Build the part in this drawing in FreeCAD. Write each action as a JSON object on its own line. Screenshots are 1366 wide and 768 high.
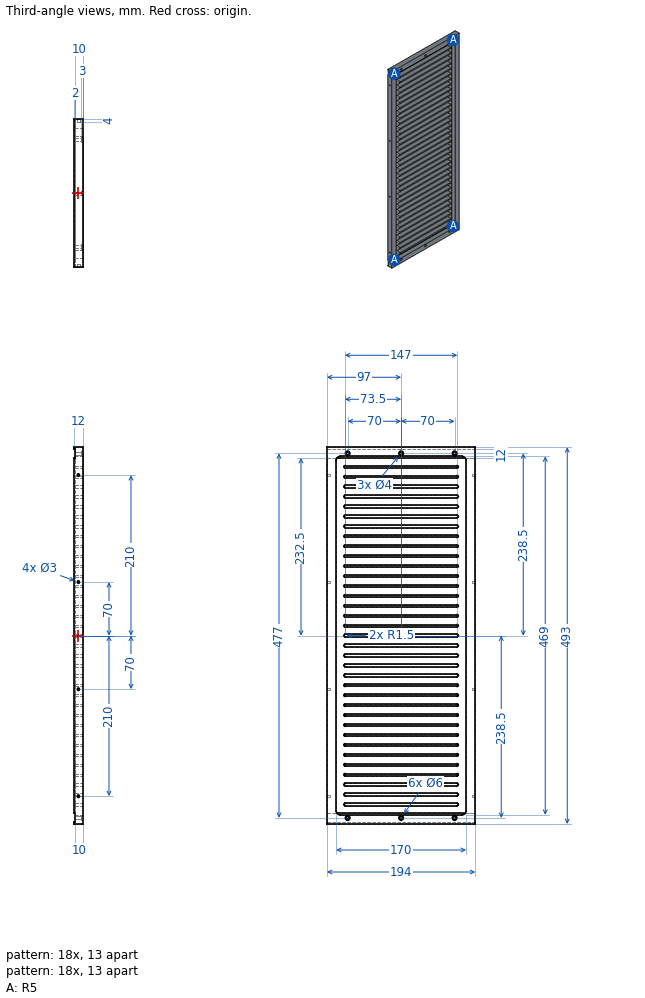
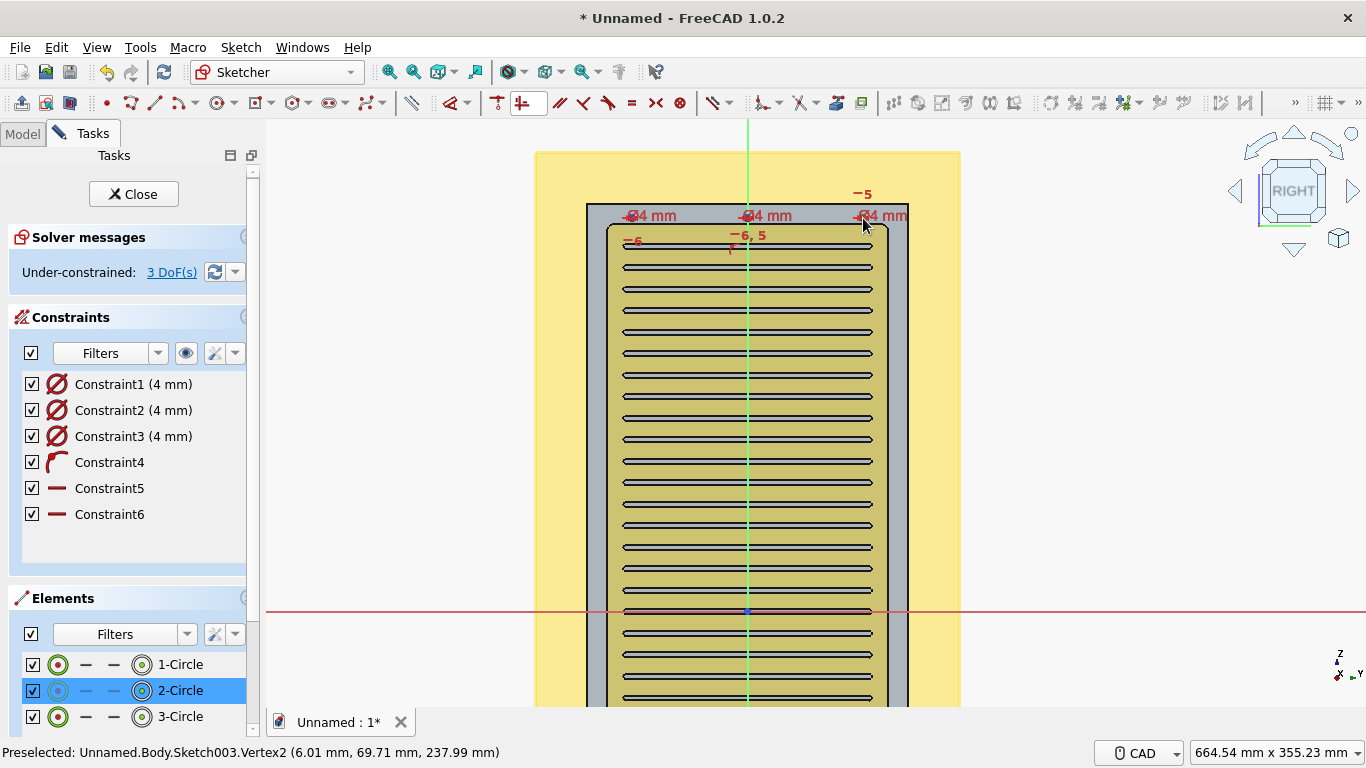
{"action": "left_click", "coordinate": [470, 104]}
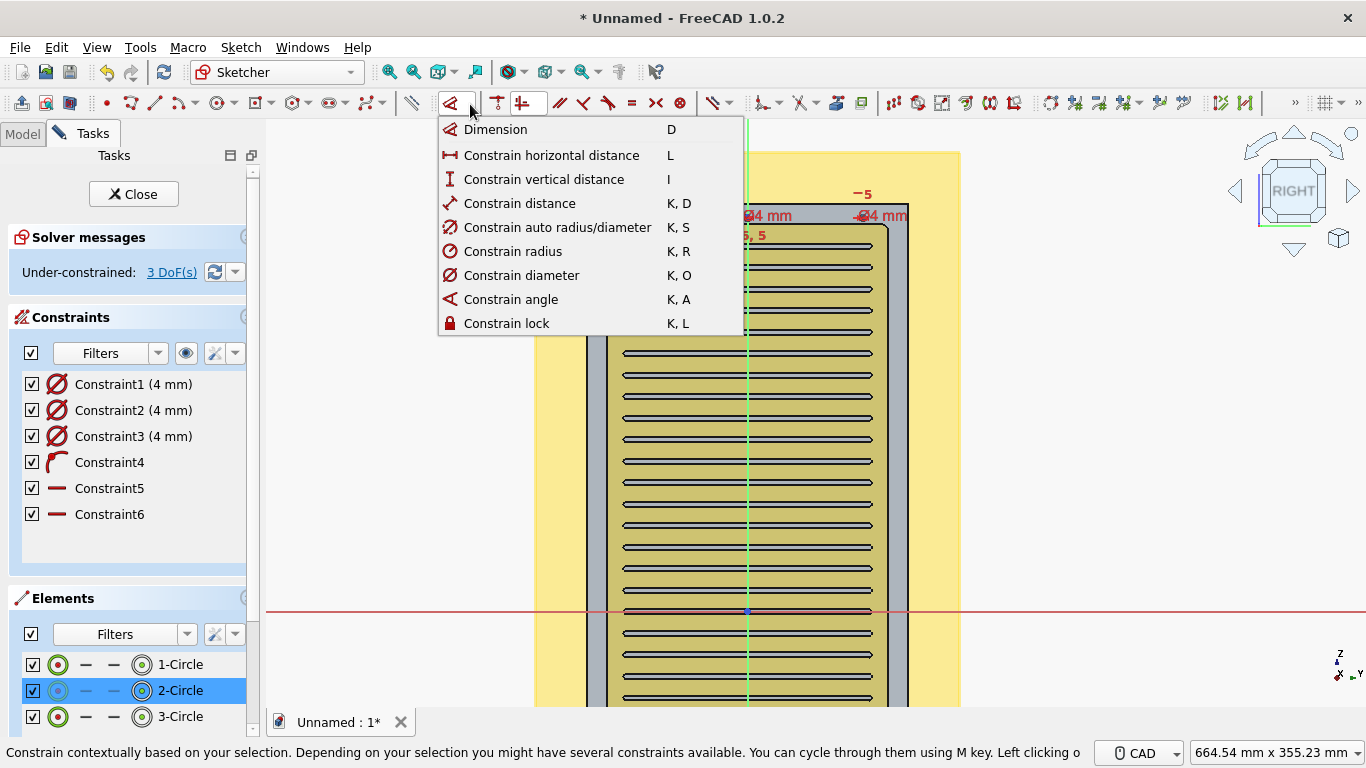
{"action": "left_click", "coordinate": [591, 155]}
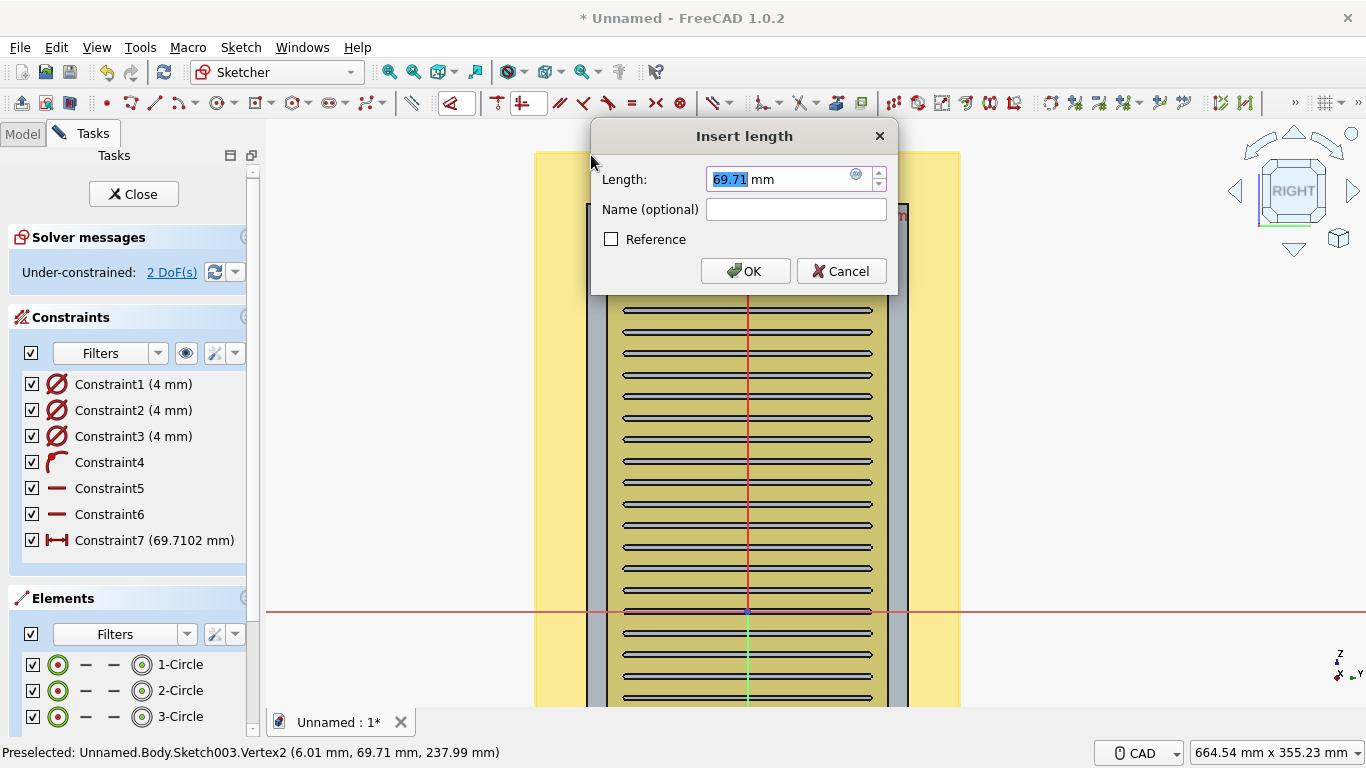
{"action": "type", "text": "70"}
{"action": "key", "text": "Return"}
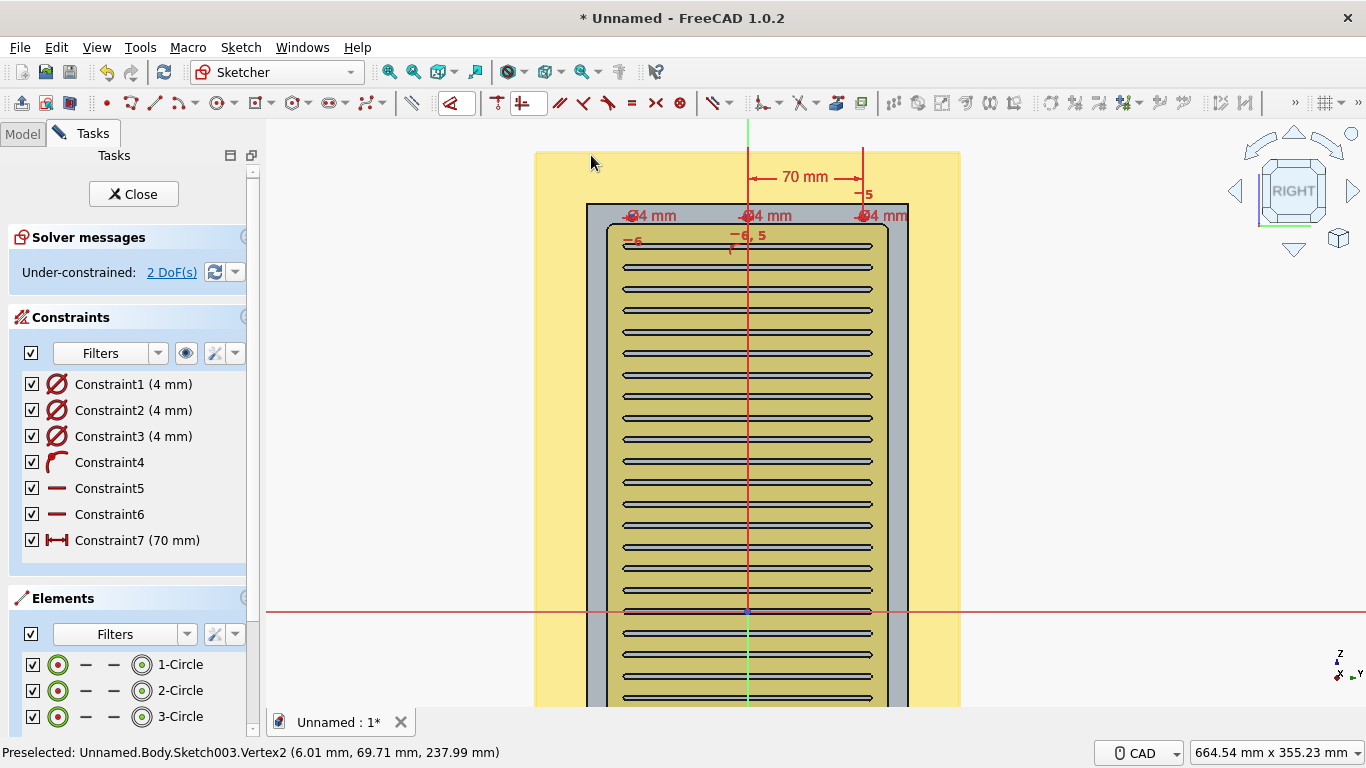
{"action": "left_click", "coordinate": [632, 218]}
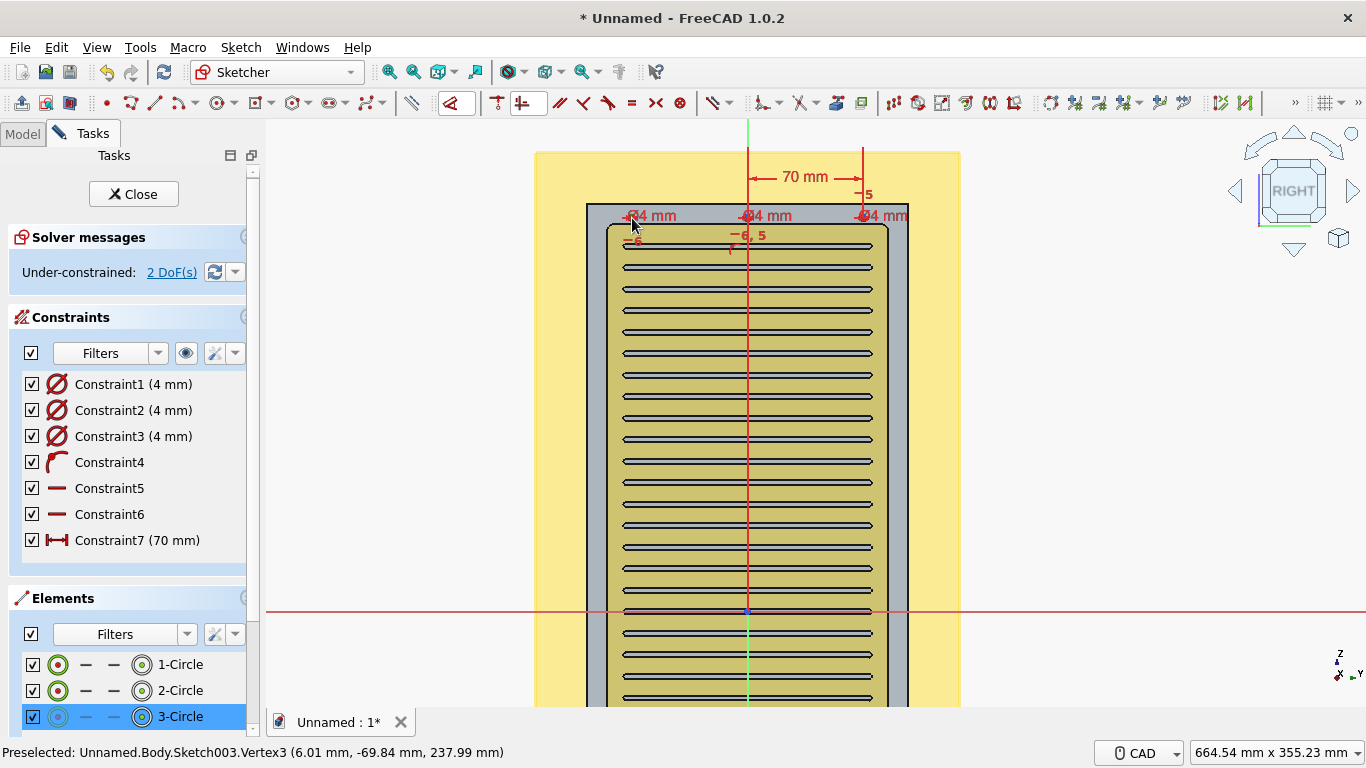
{"action": "key", "text": "l"}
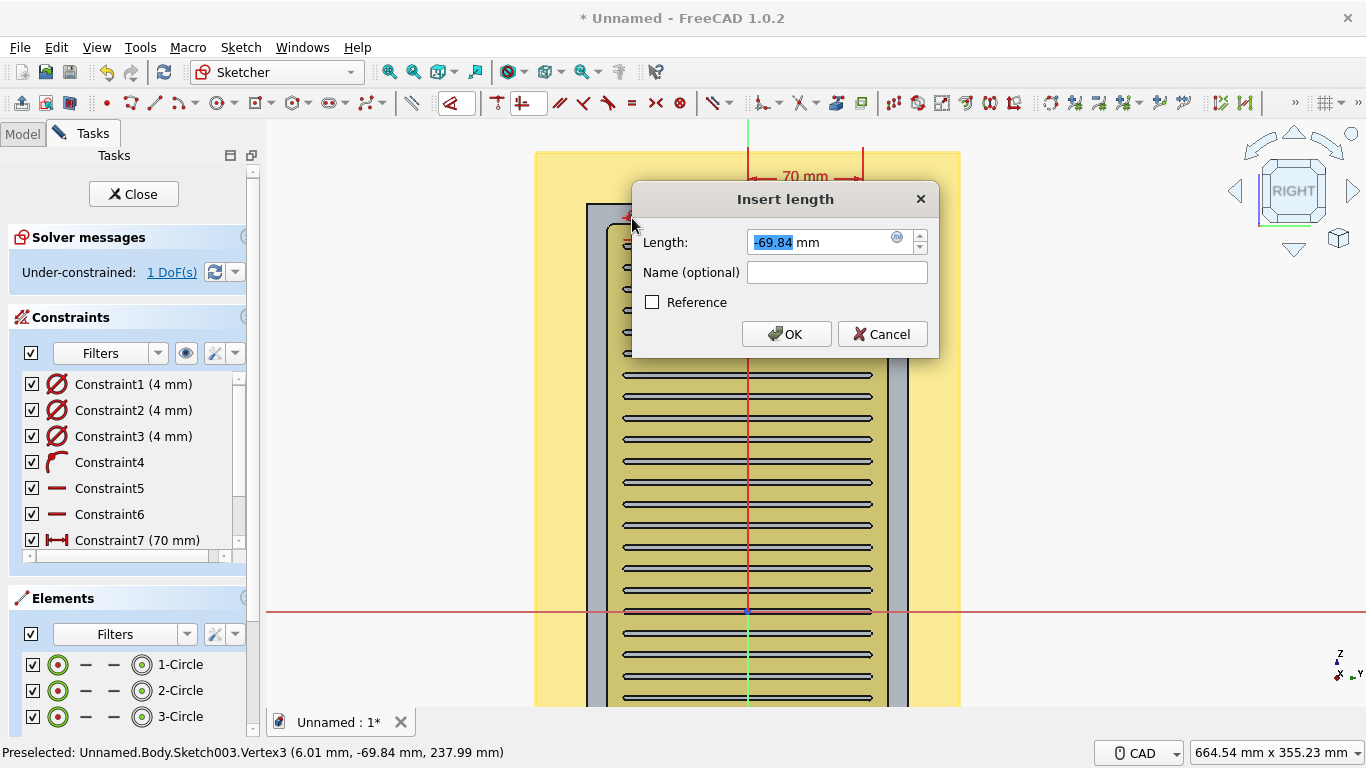
{"action": "type", "text": "-70"}
{"action": "key", "text": "Return"}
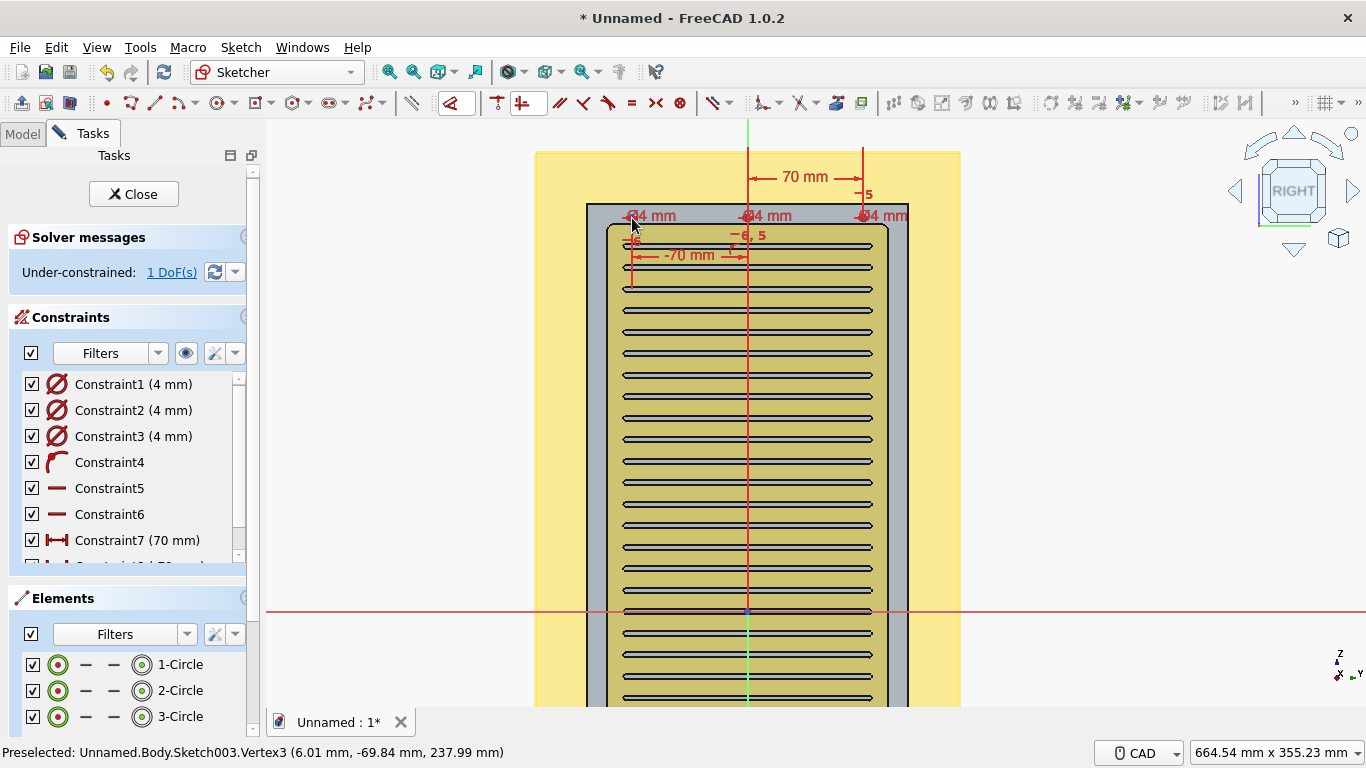
{"action": "left_click", "coordinate": [748, 218]}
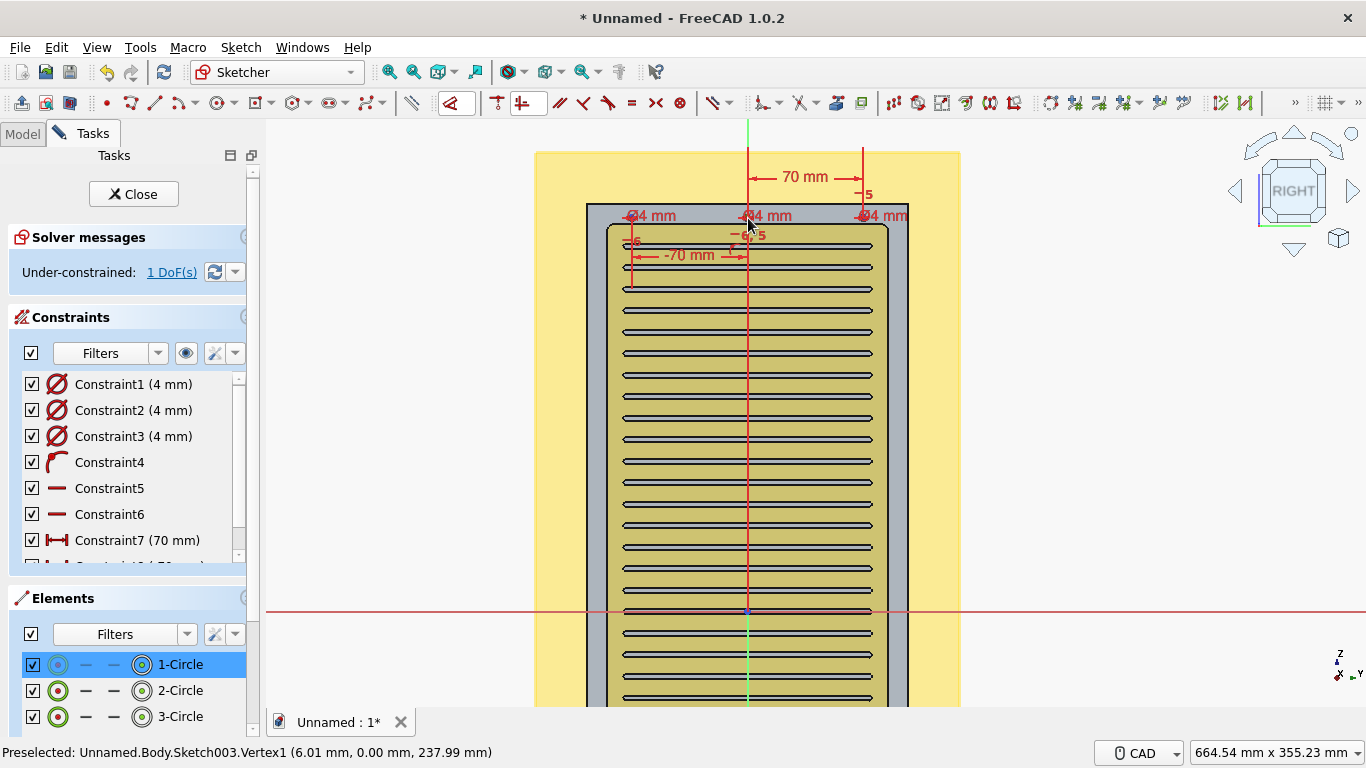
{"action": "key", "text": "i"}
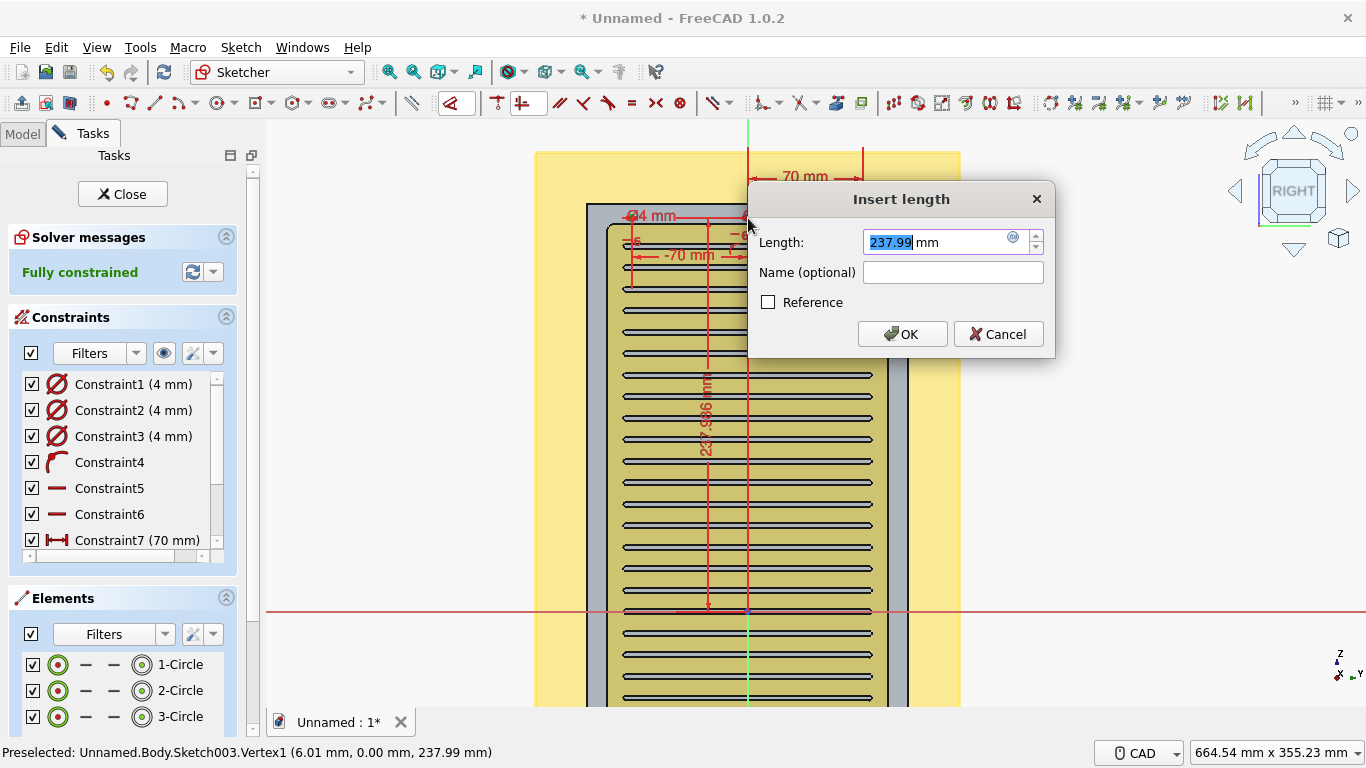
{"action": "type", "text": "238.5"}
{"action": "key", "text": "Return"}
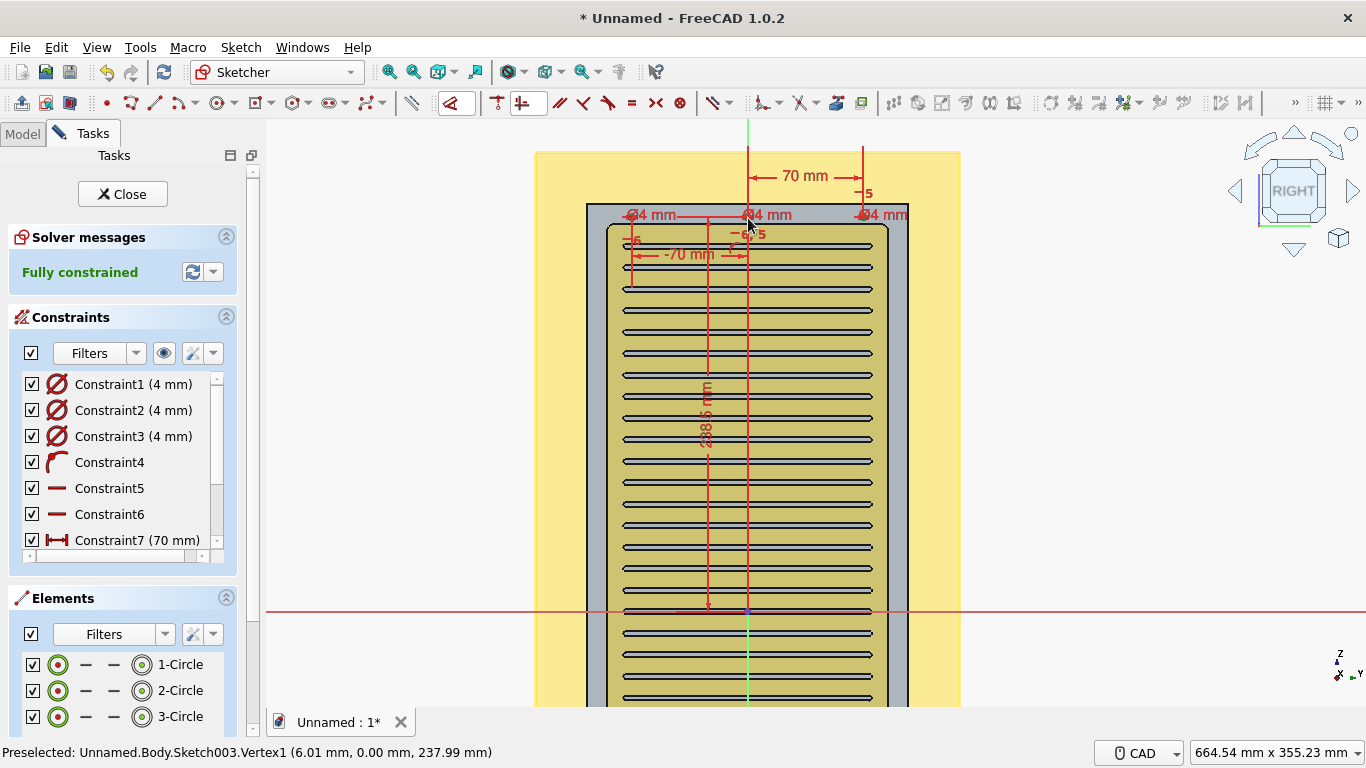
{"action": "left_click", "coordinate": [123, 194]}